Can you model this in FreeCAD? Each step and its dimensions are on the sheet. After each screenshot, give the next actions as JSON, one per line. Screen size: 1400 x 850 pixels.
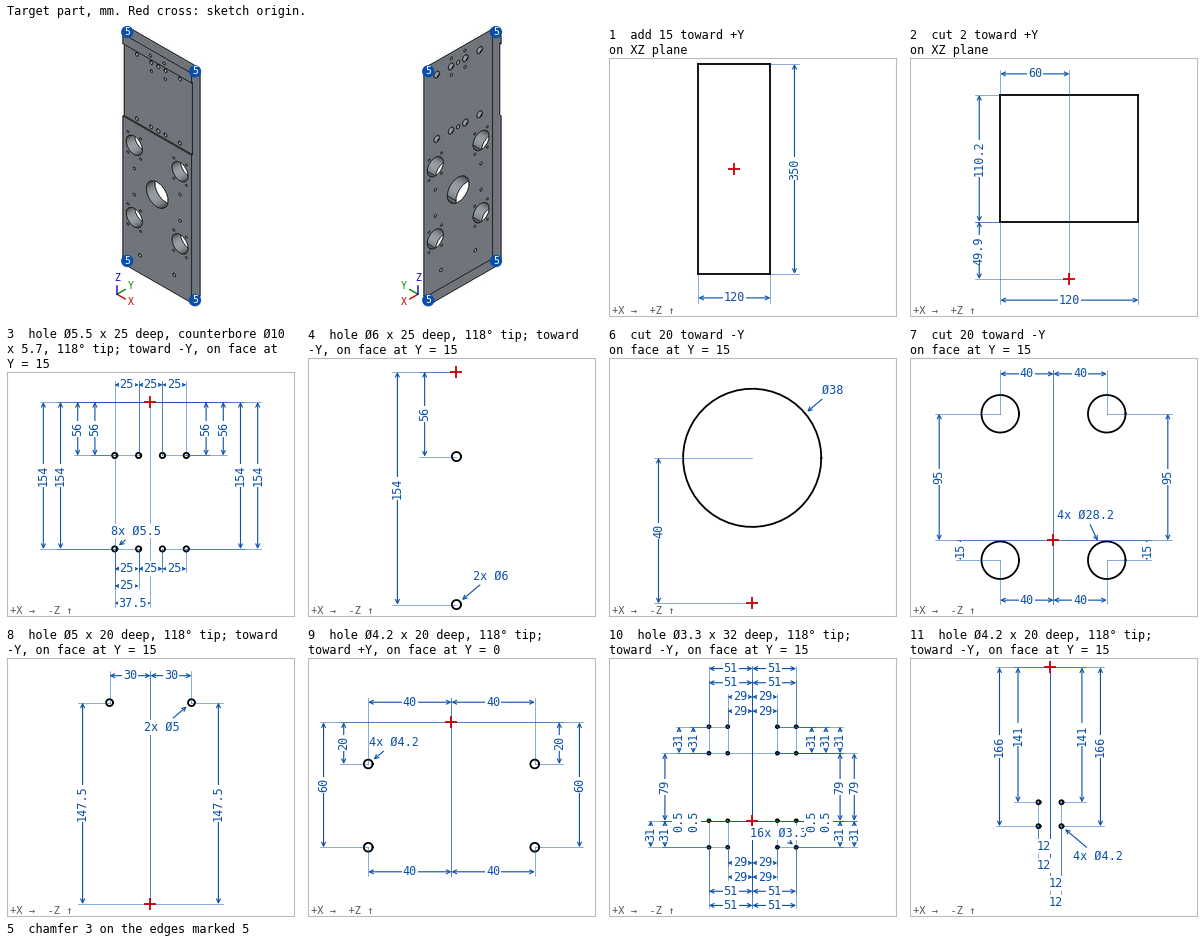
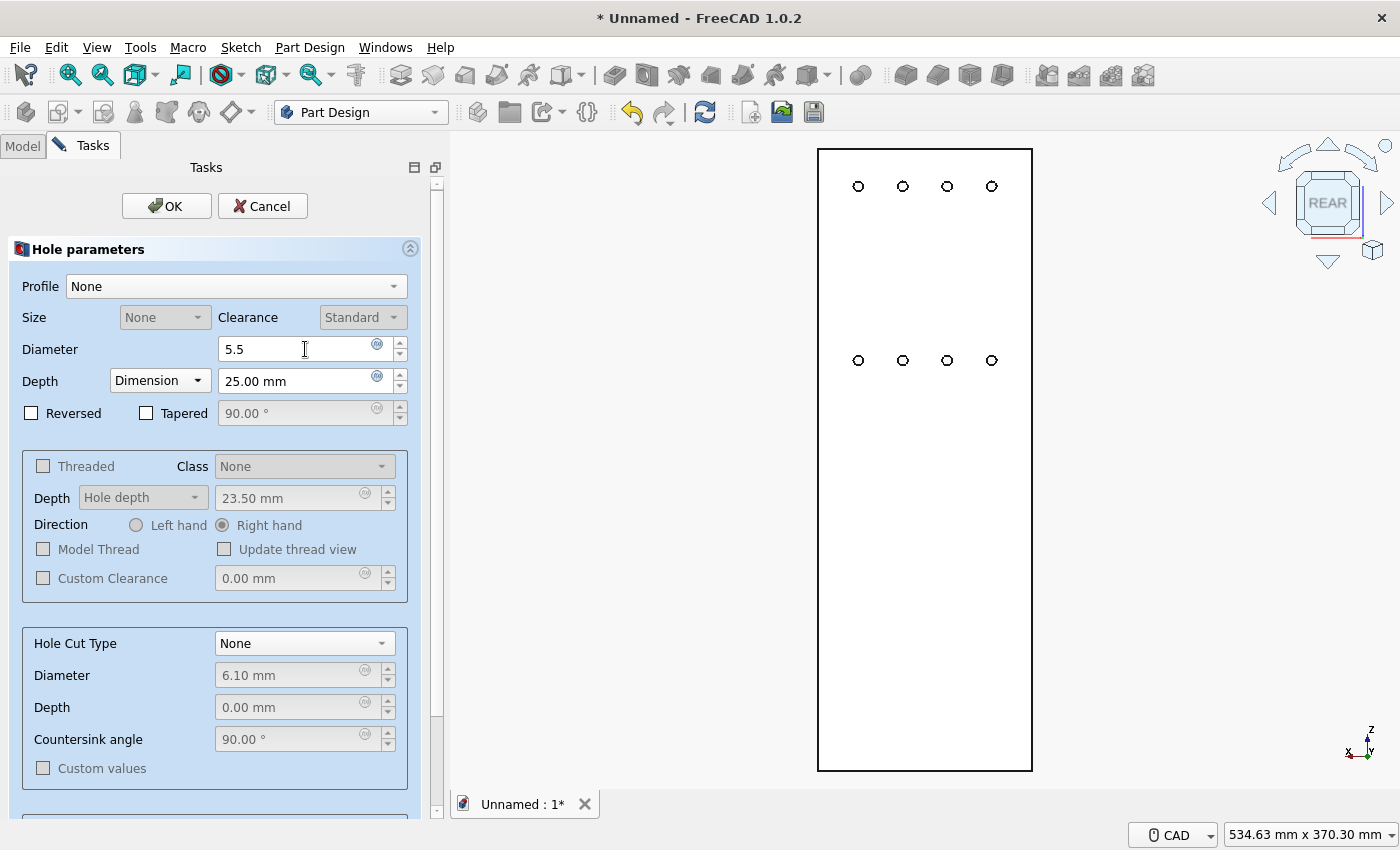
{"action": "triple_click", "coordinate": [305, 381]}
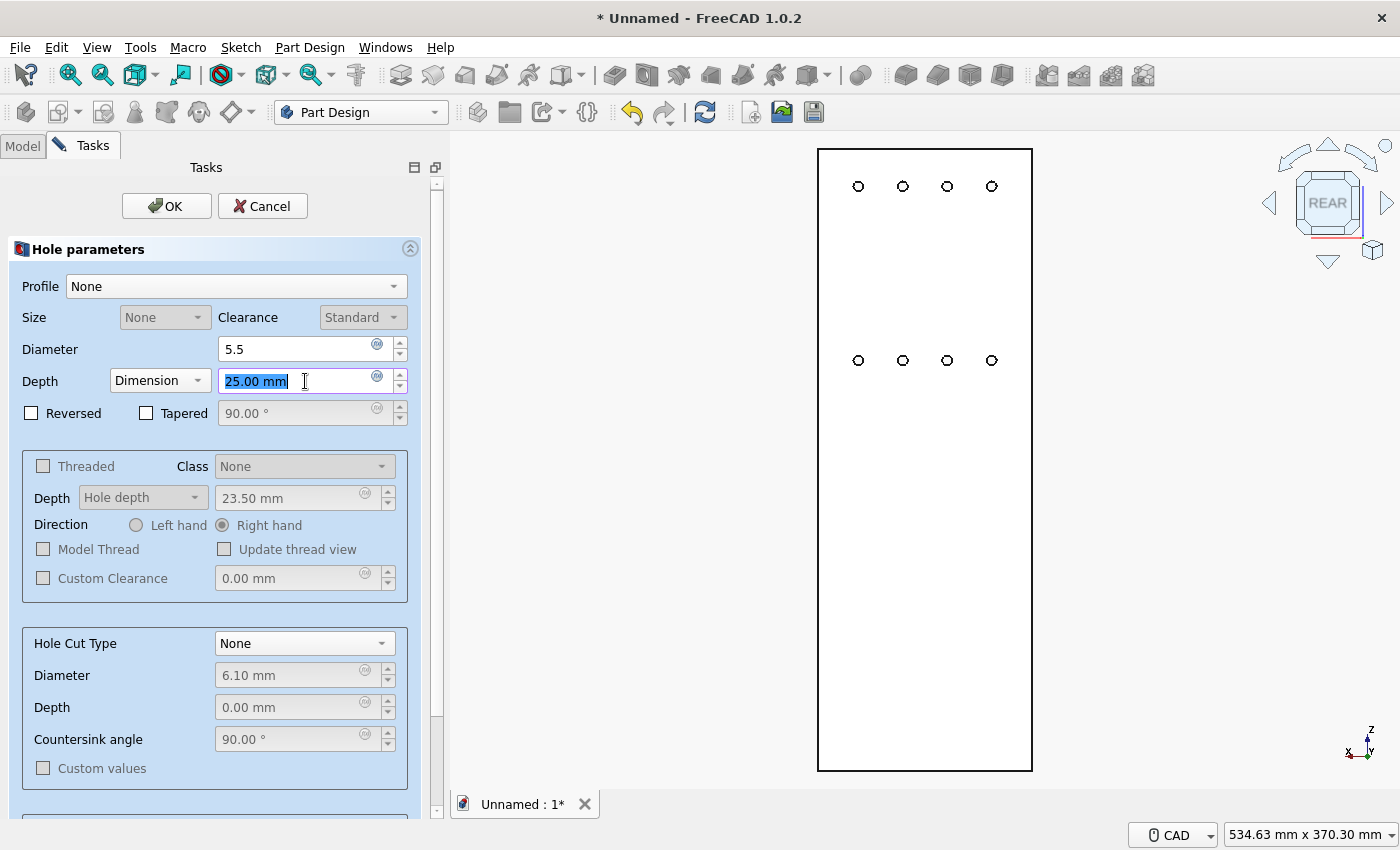
{"action": "type", "text": "25"}
{"action": "key", "text": "Tab"}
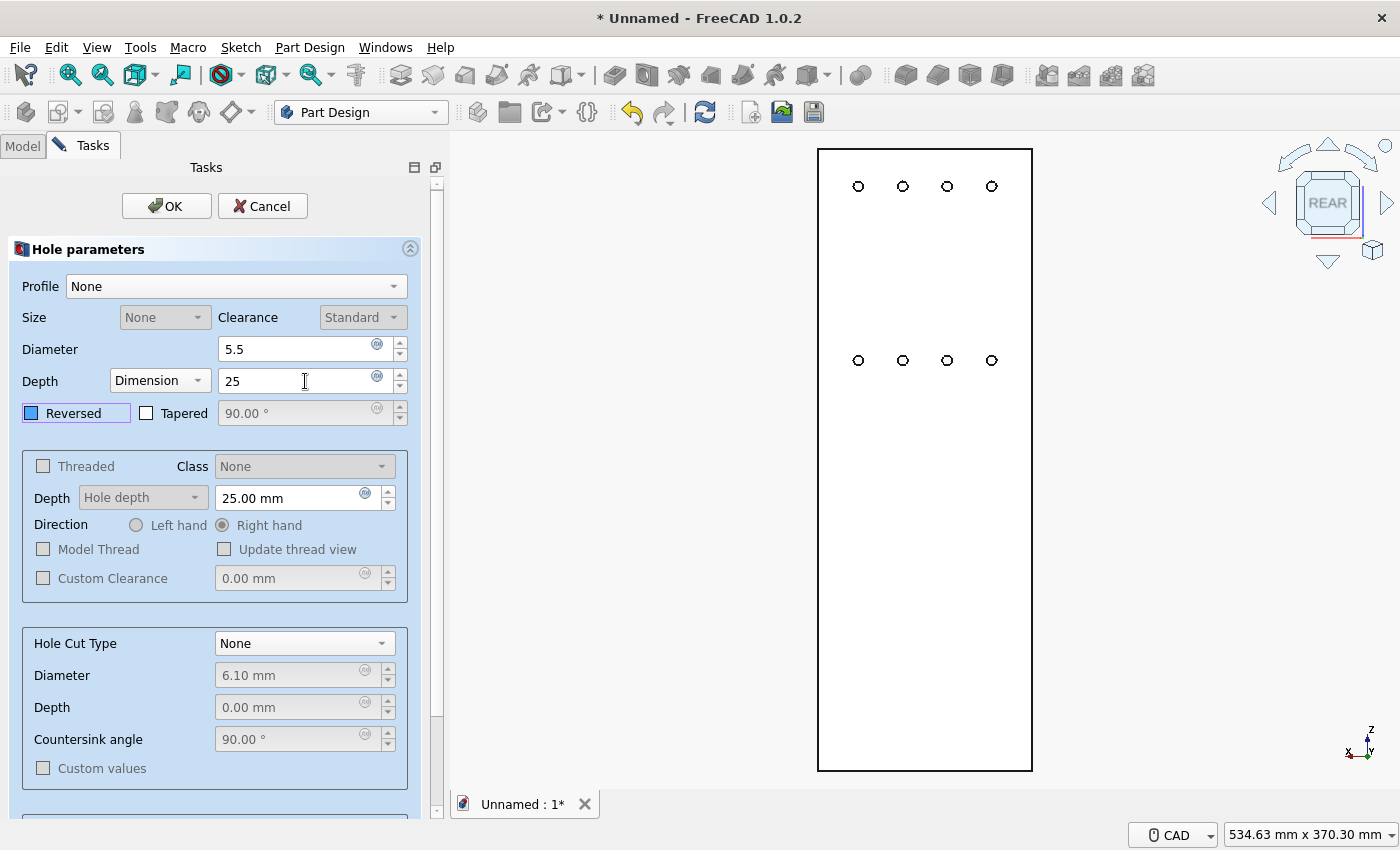
{"action": "left_click", "coordinate": [306, 644]}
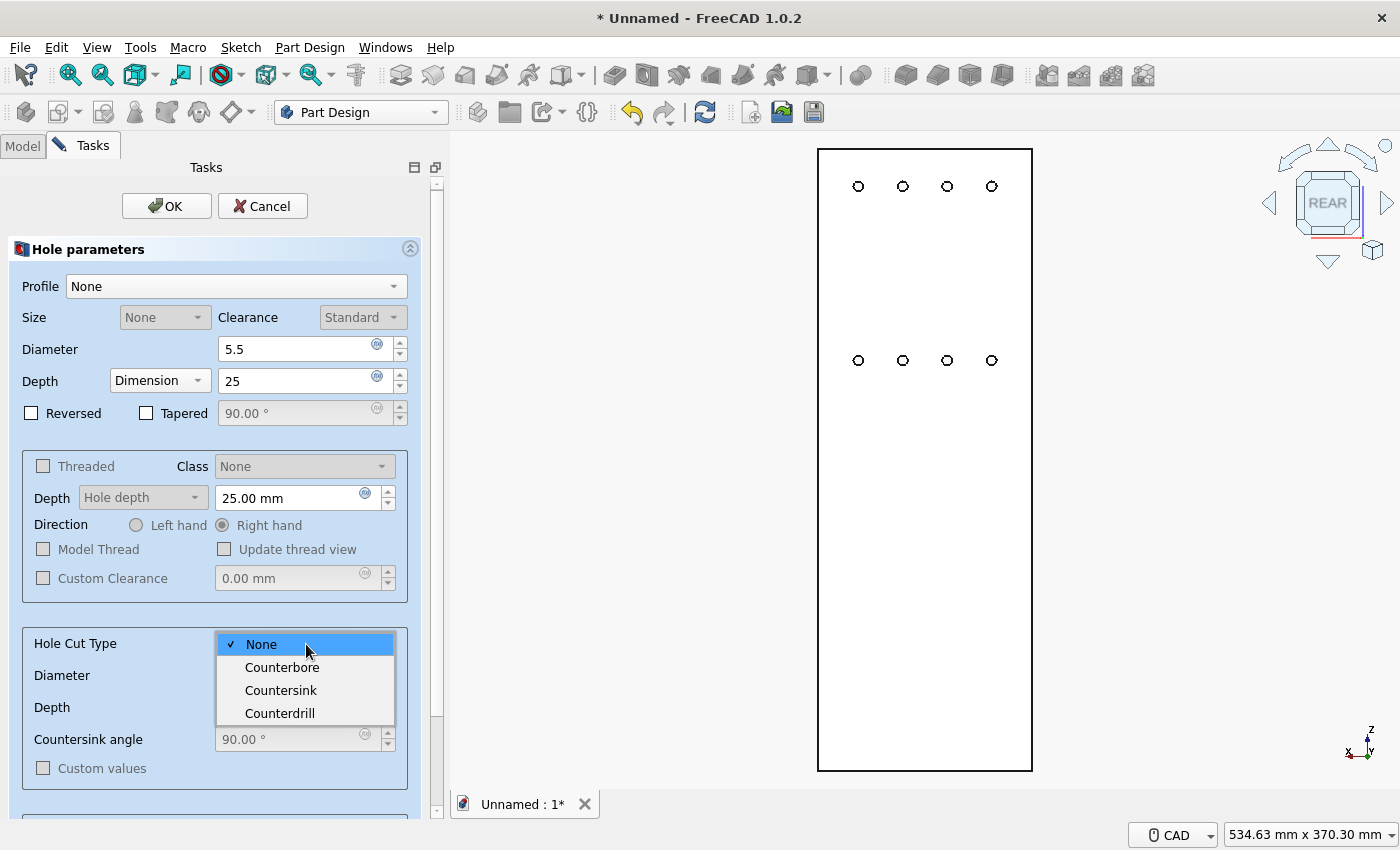
{"action": "left_click", "coordinate": [304, 668]}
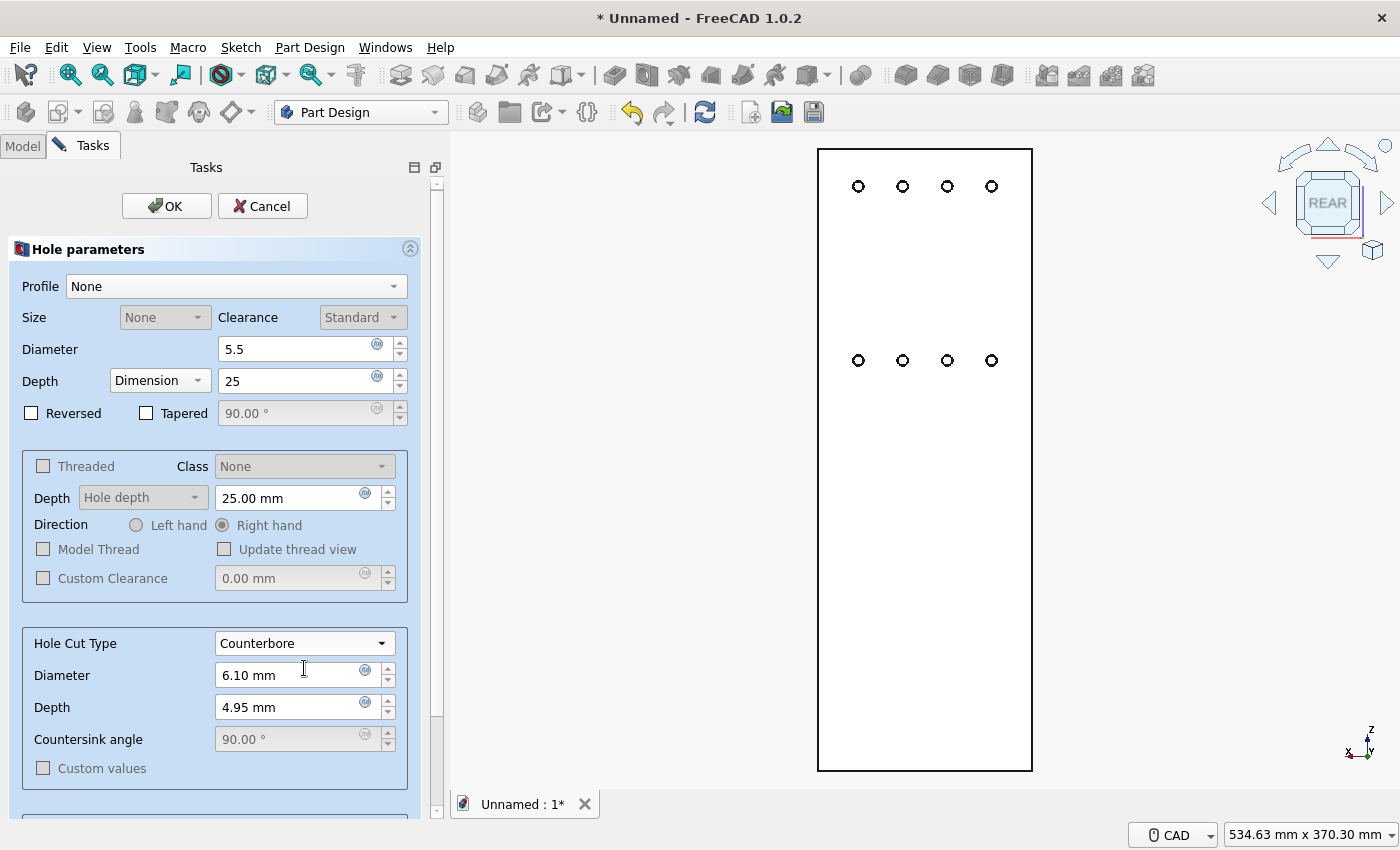
{"action": "triple_click", "coordinate": [298, 675]}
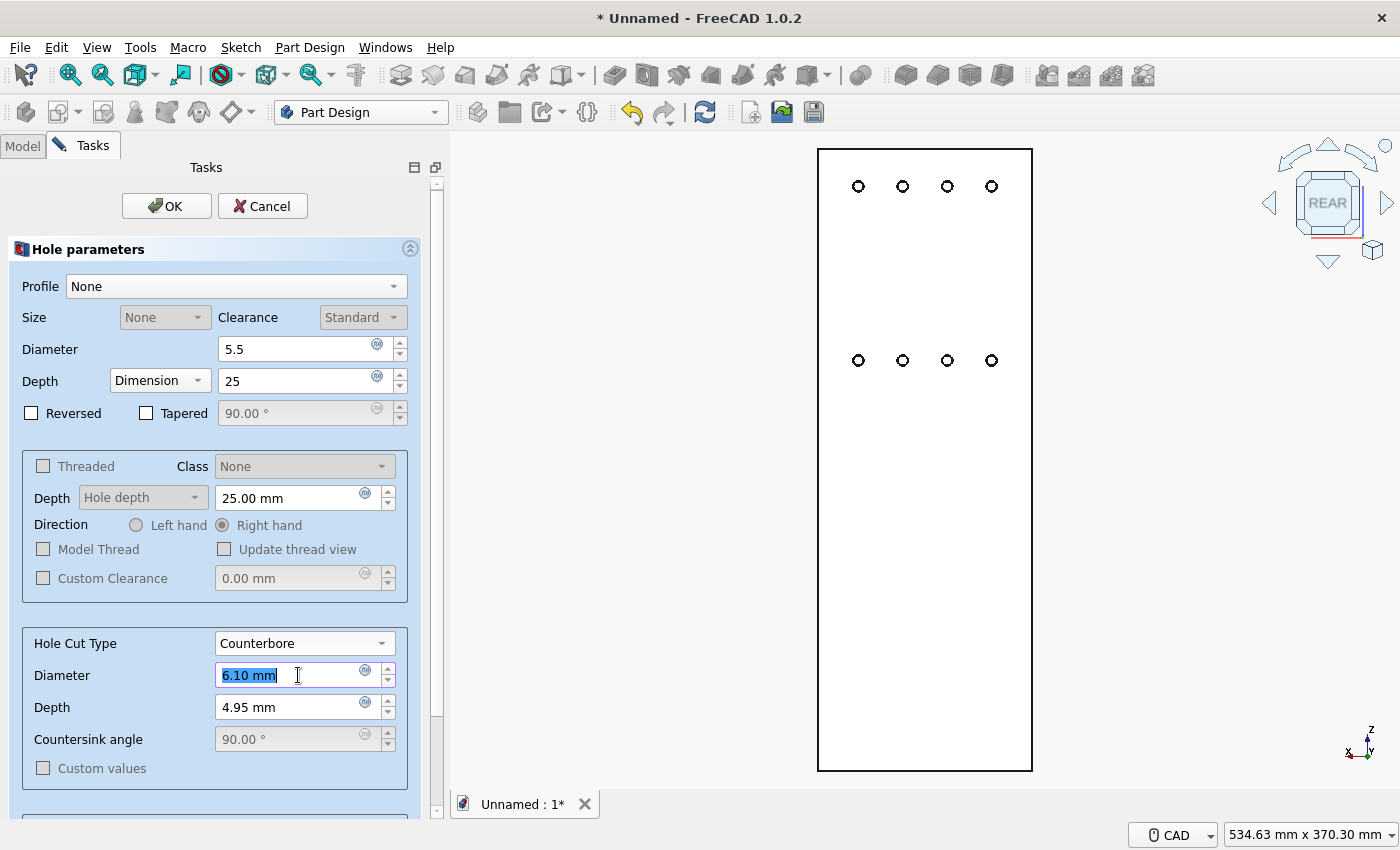
{"action": "type", "text": "10"}
{"action": "key", "text": "Tab"}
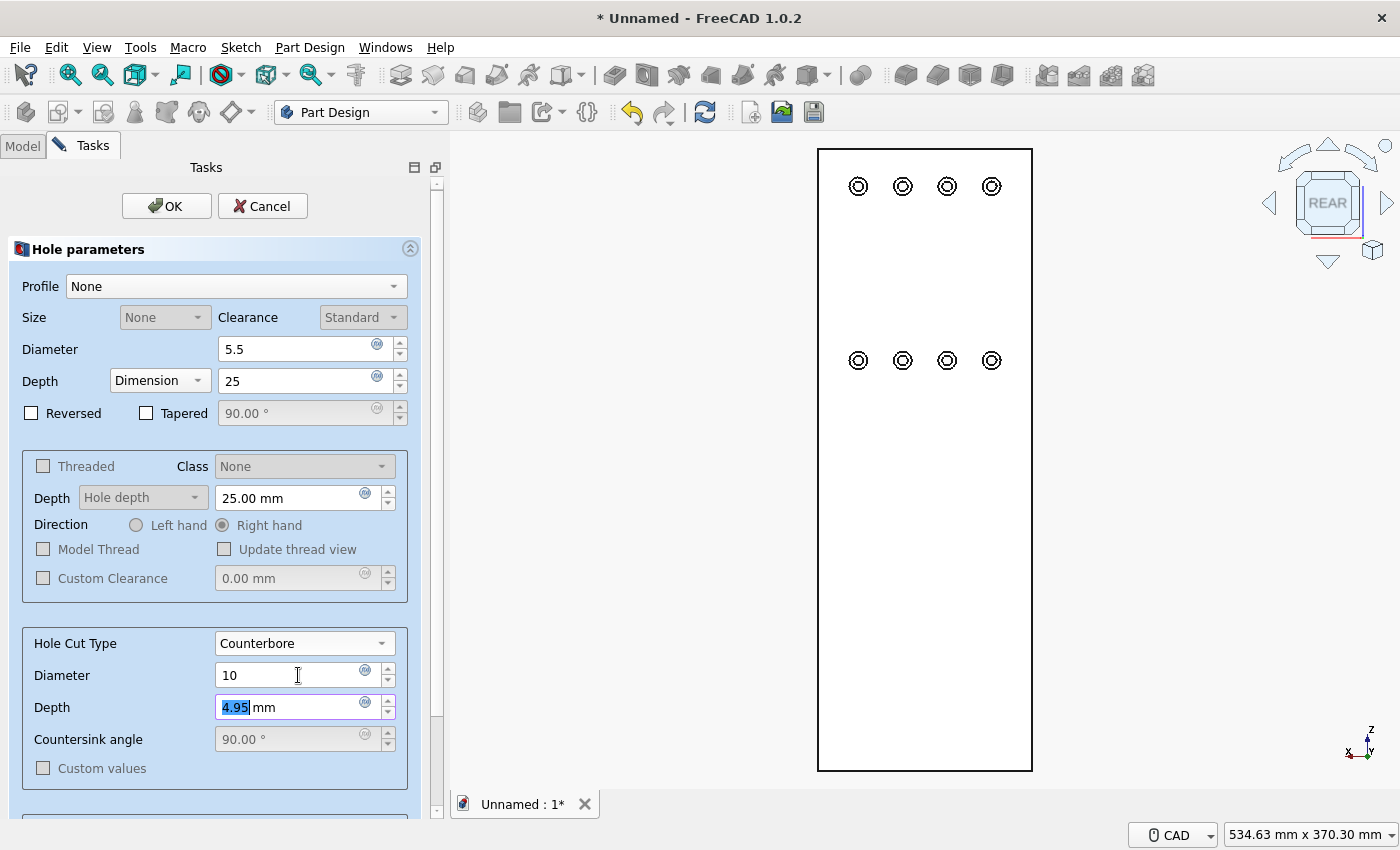
{"action": "type", "text": "5.7"}
{"action": "key", "text": "Tab"}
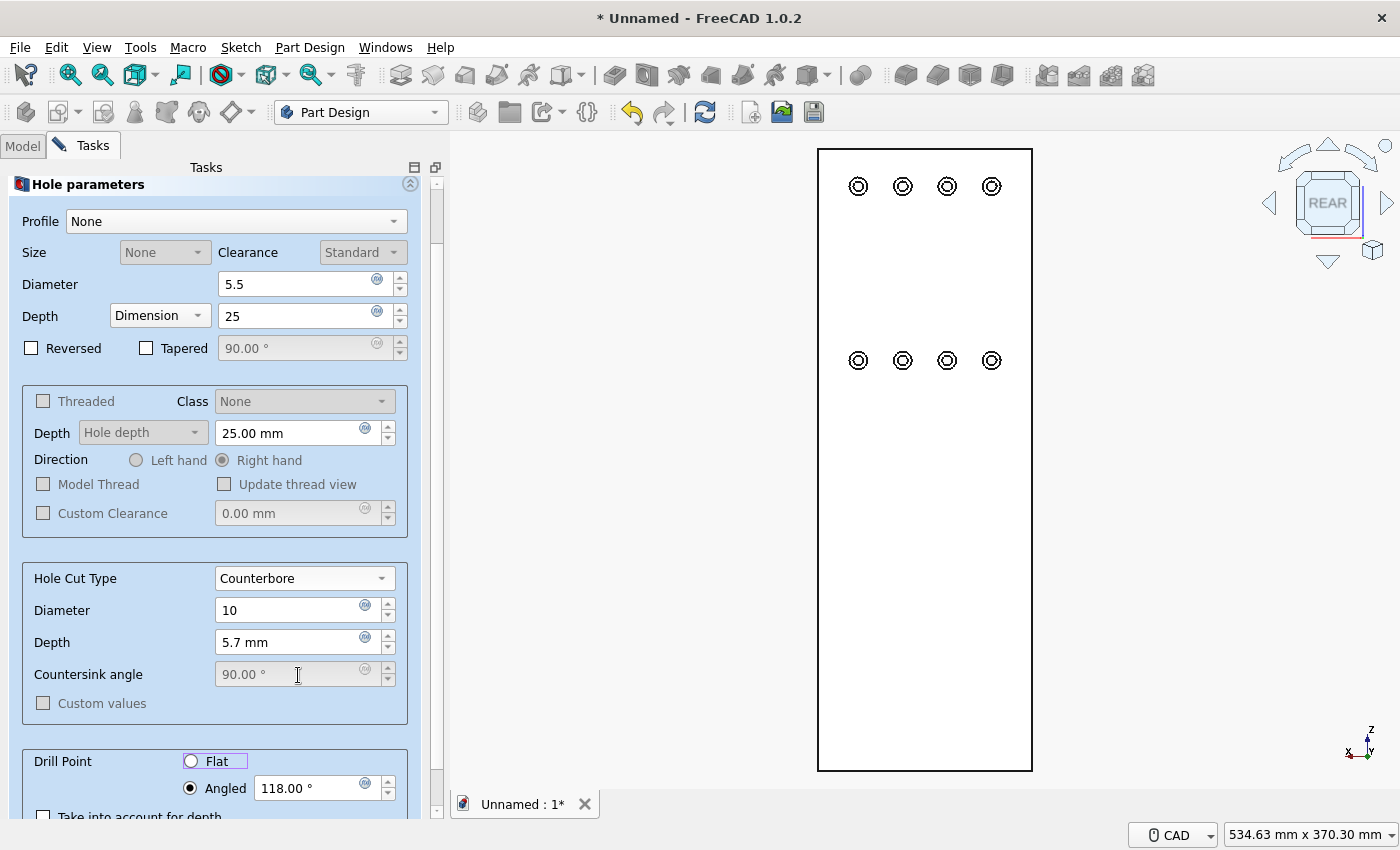
{"action": "scroll", "coordinate": [437, 498], "scroll_direction": "up", "scroll_amount": 2}